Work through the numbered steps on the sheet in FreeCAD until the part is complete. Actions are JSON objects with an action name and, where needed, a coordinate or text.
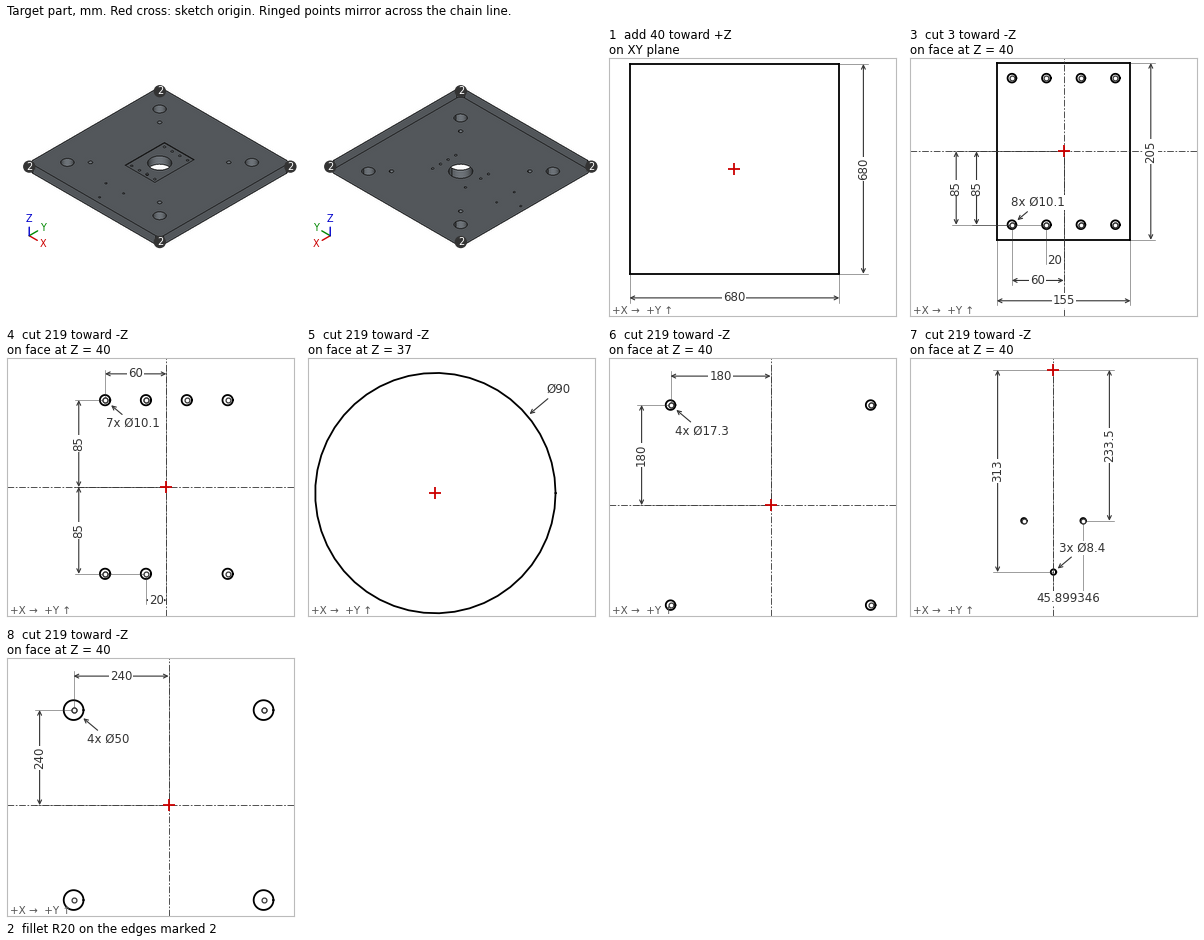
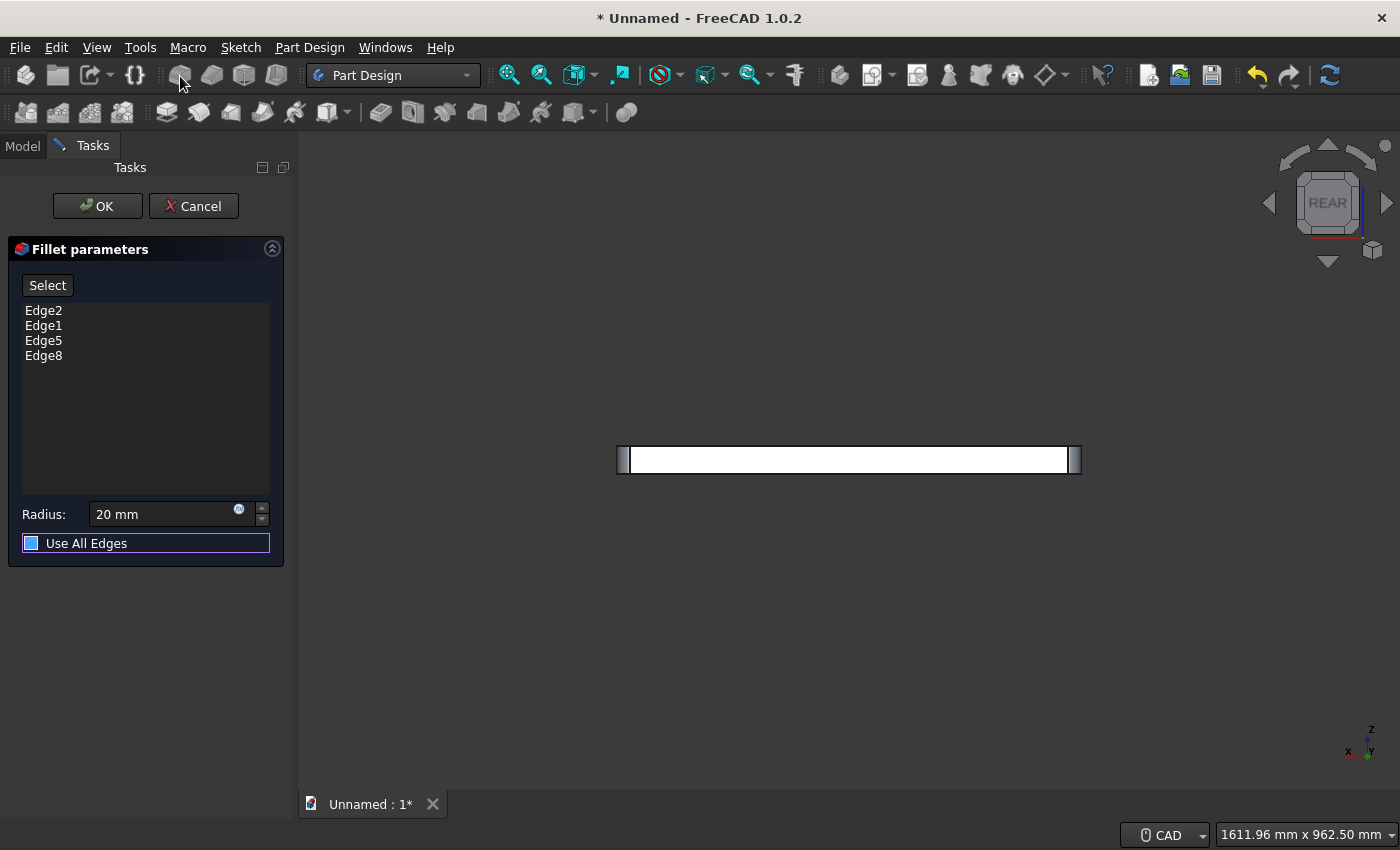
{"action": "left_click", "coordinate": [98, 206]}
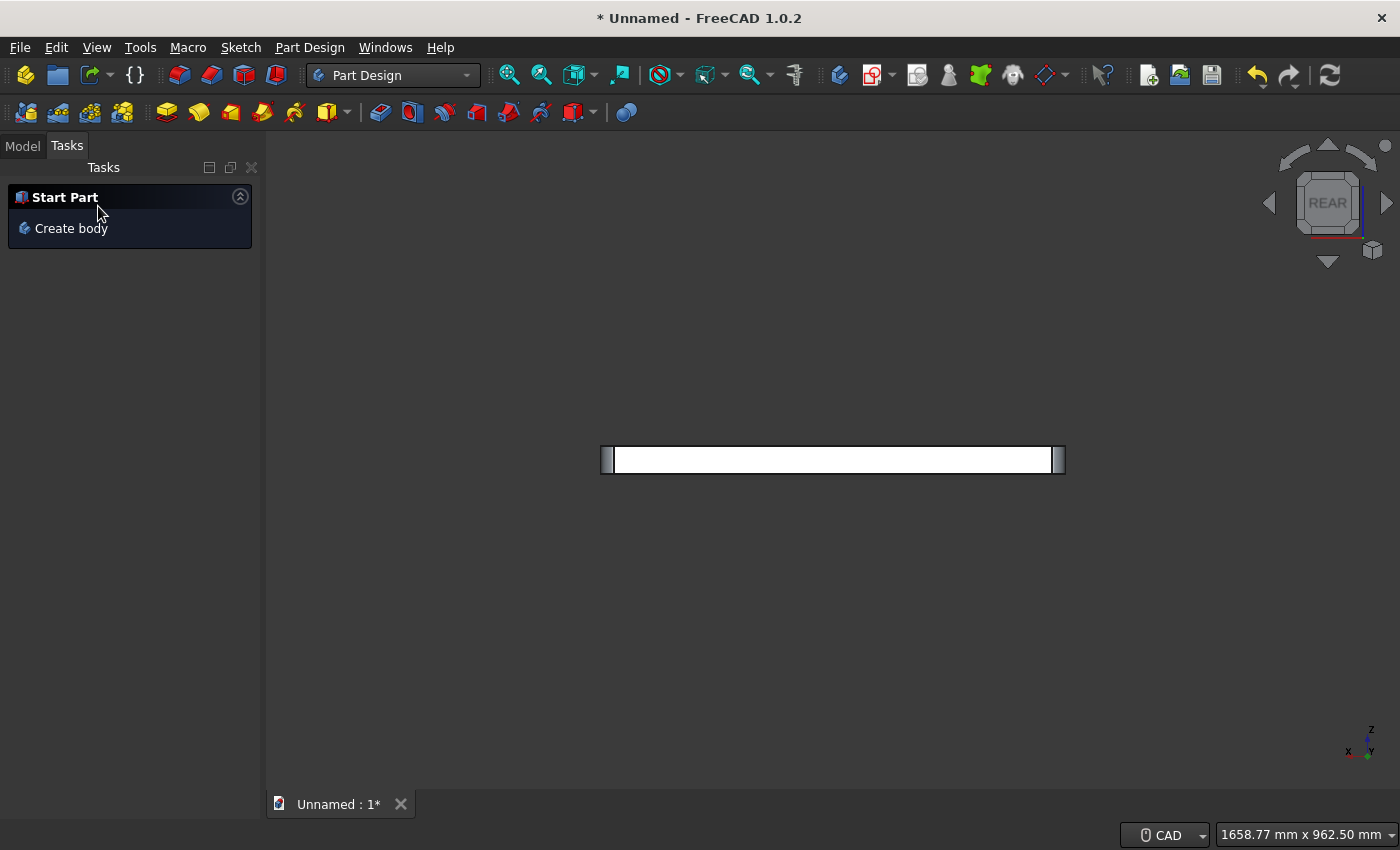
{"action": "left_click", "coordinate": [510, 76]}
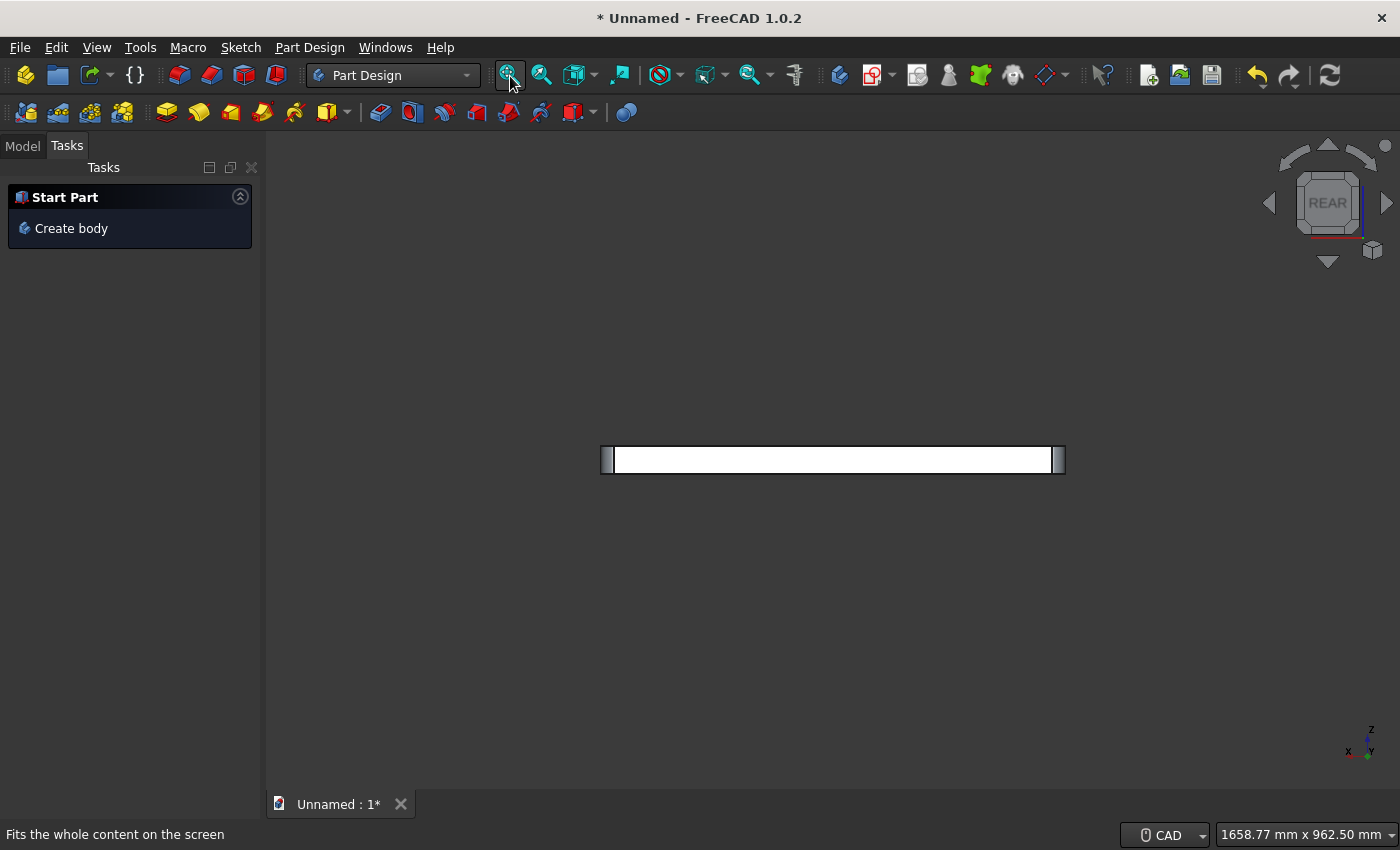
{"action": "key", "text": "0"}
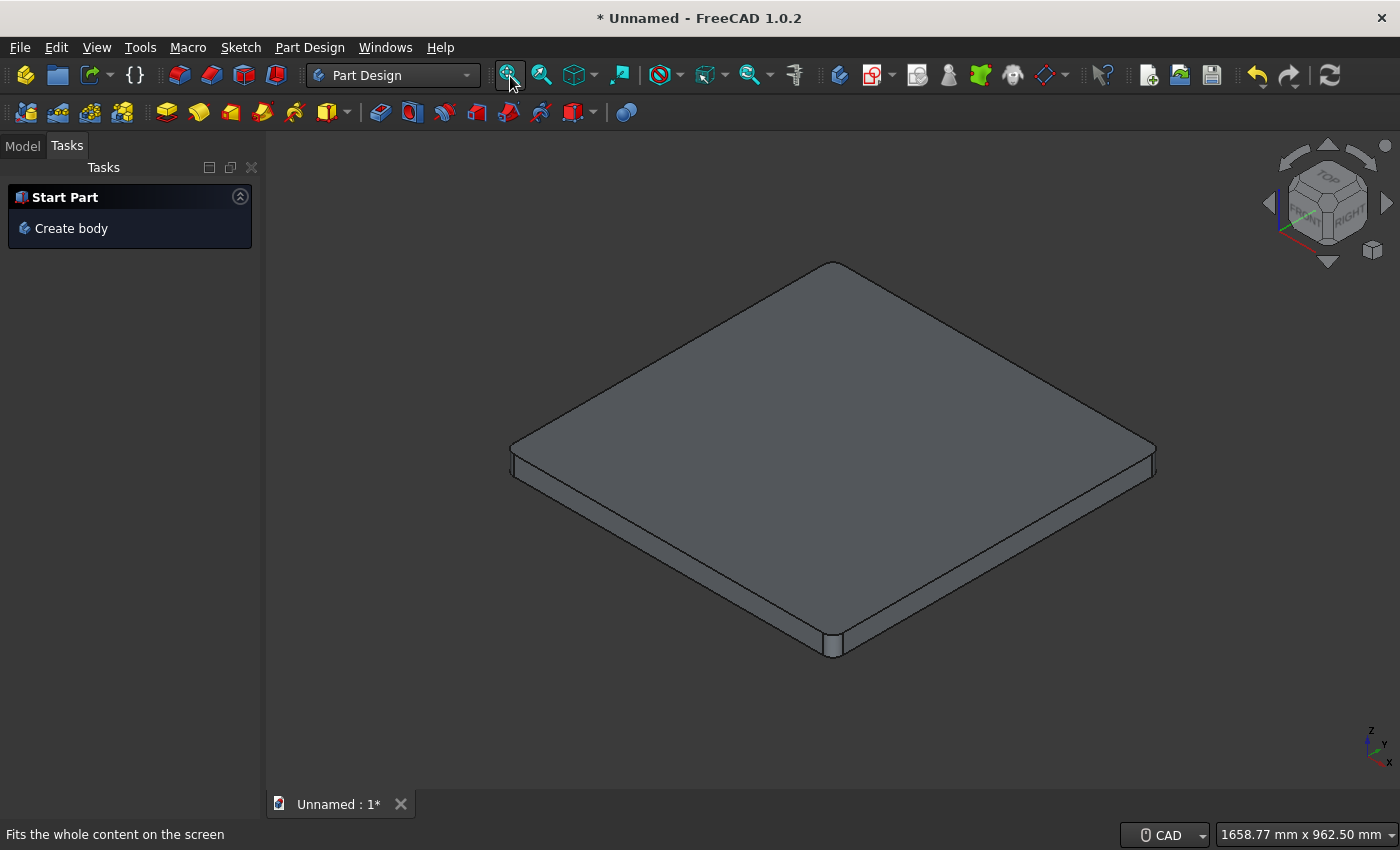
{"action": "left_click", "coordinate": [833, 448]}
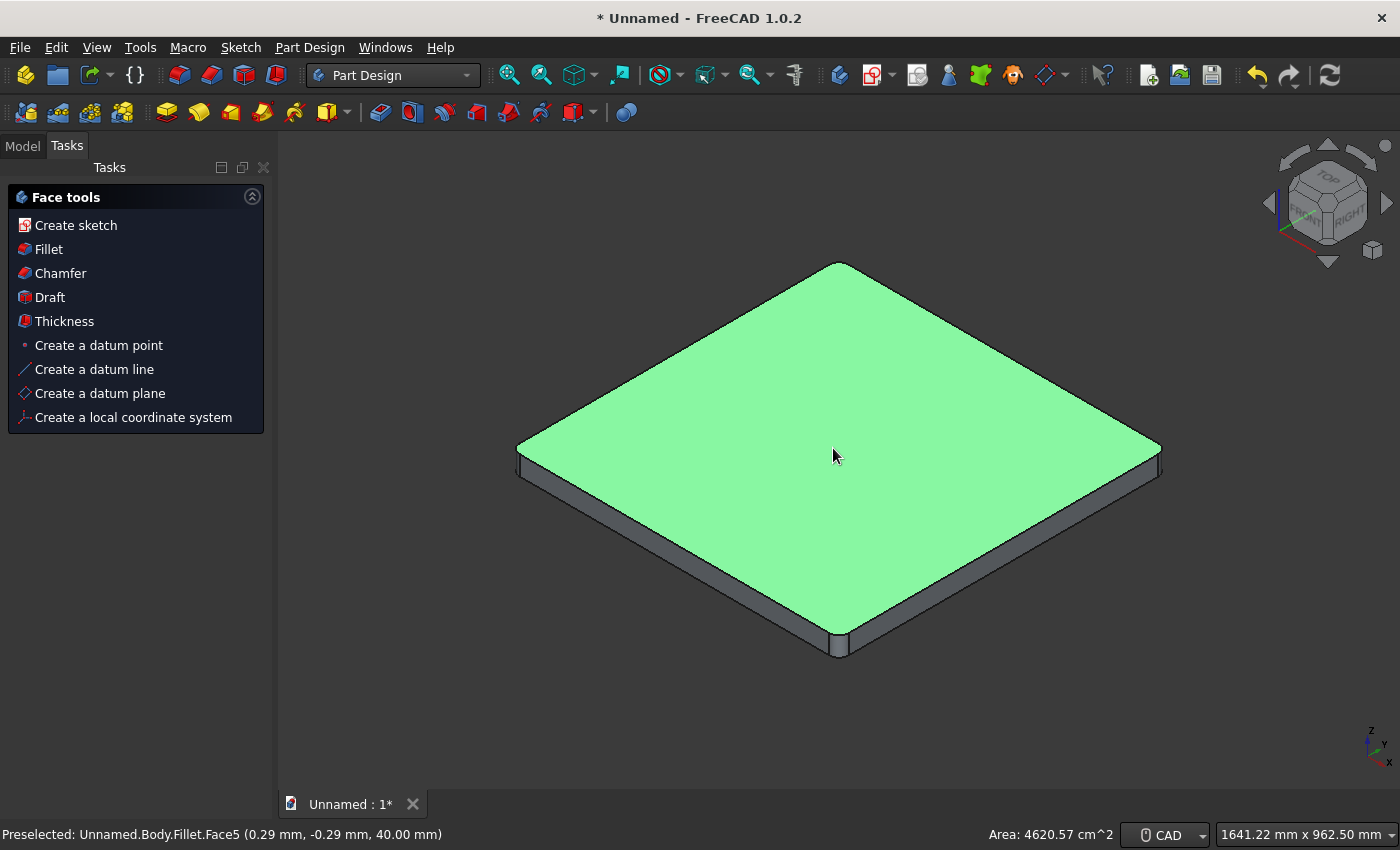
{"action": "left_click", "coordinate": [872, 76]}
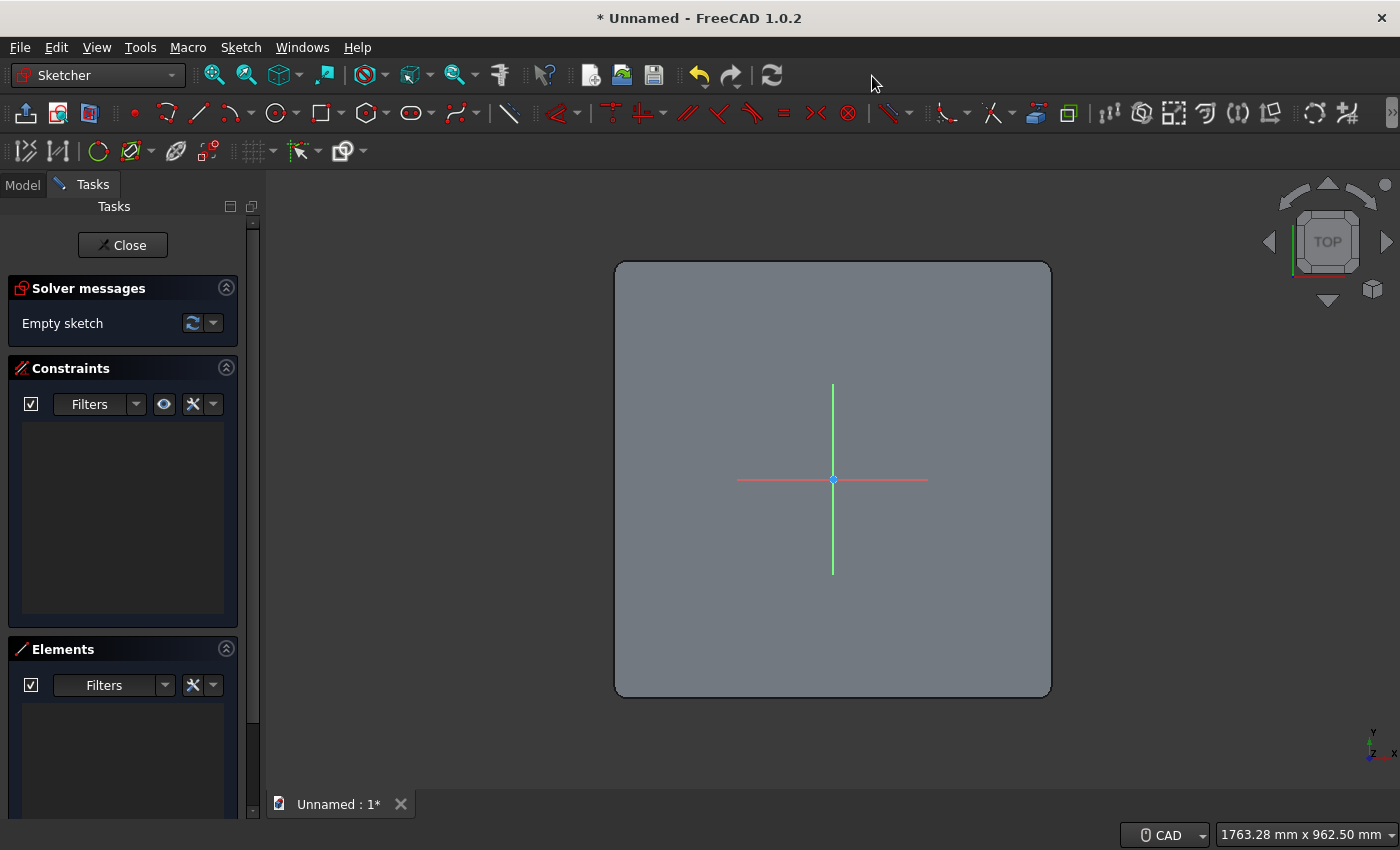
{"action": "scroll", "coordinate": [863, 480], "scroll_direction": "up", "scroll_amount": 6}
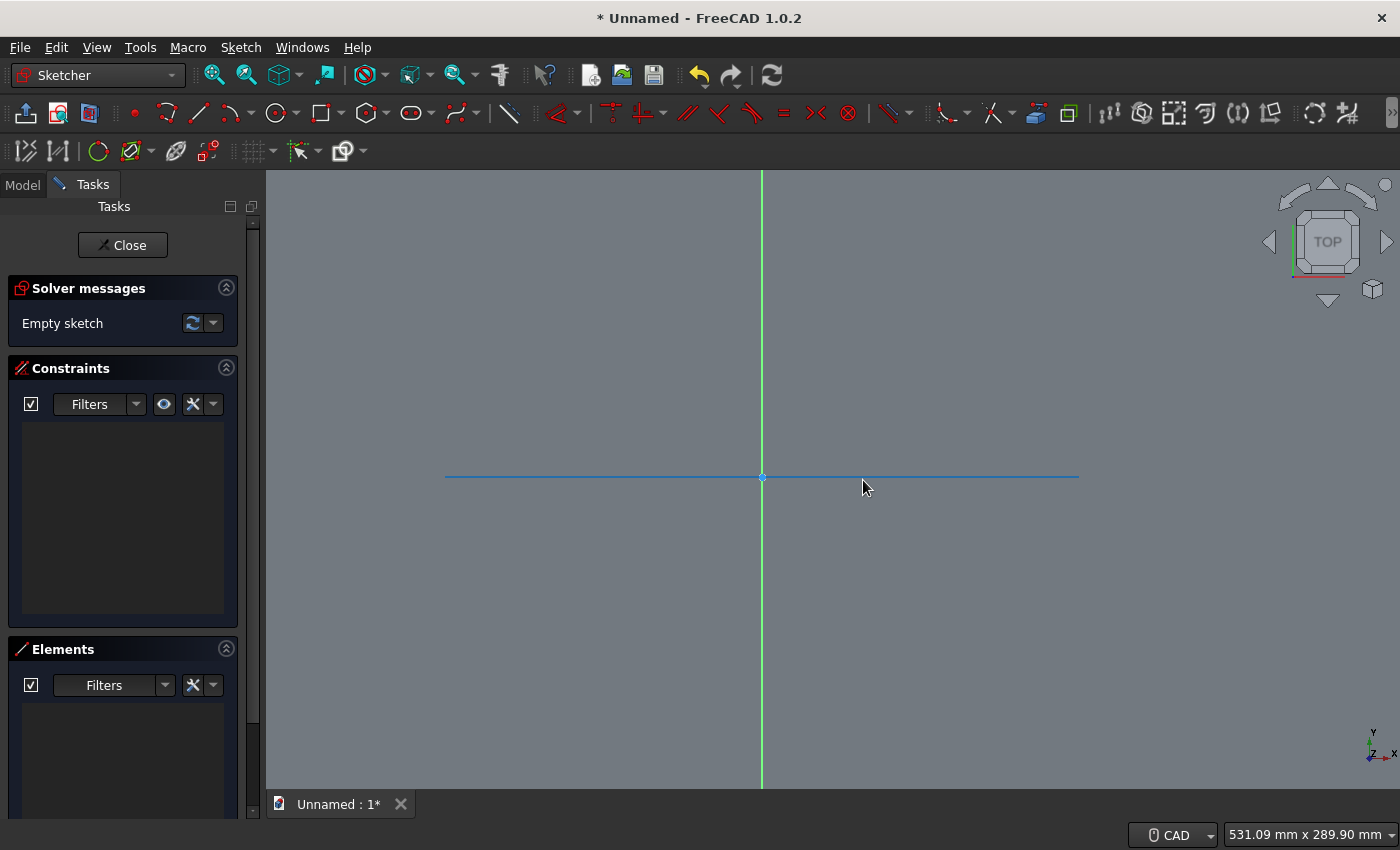
{"action": "key", "text": "g v"}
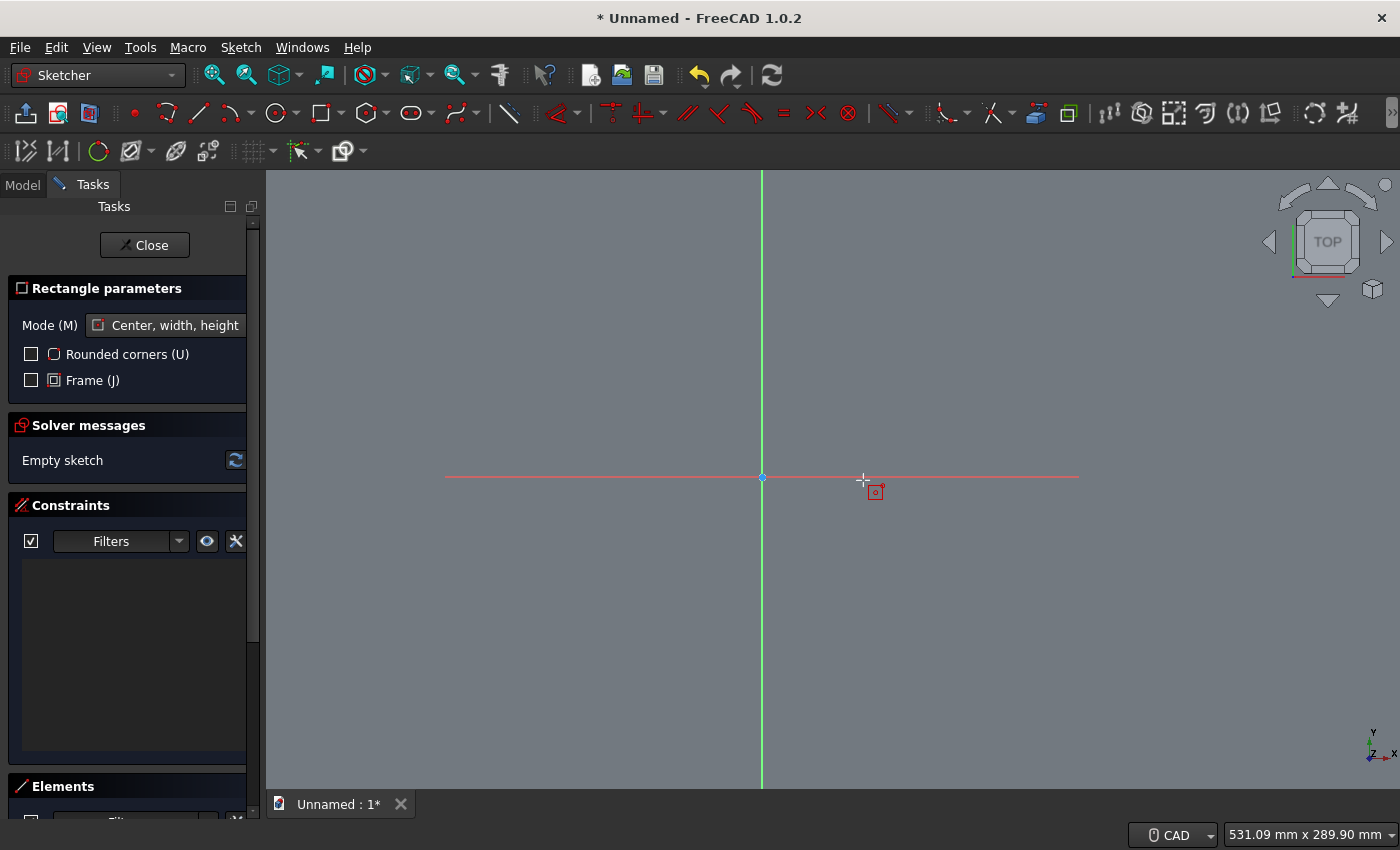
{"action": "left_click", "coordinate": [762, 477]}
{"action": "left_click", "coordinate": [928, 258]}